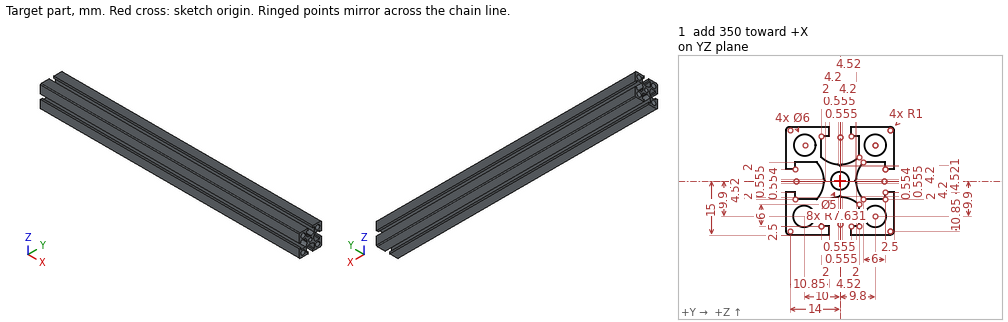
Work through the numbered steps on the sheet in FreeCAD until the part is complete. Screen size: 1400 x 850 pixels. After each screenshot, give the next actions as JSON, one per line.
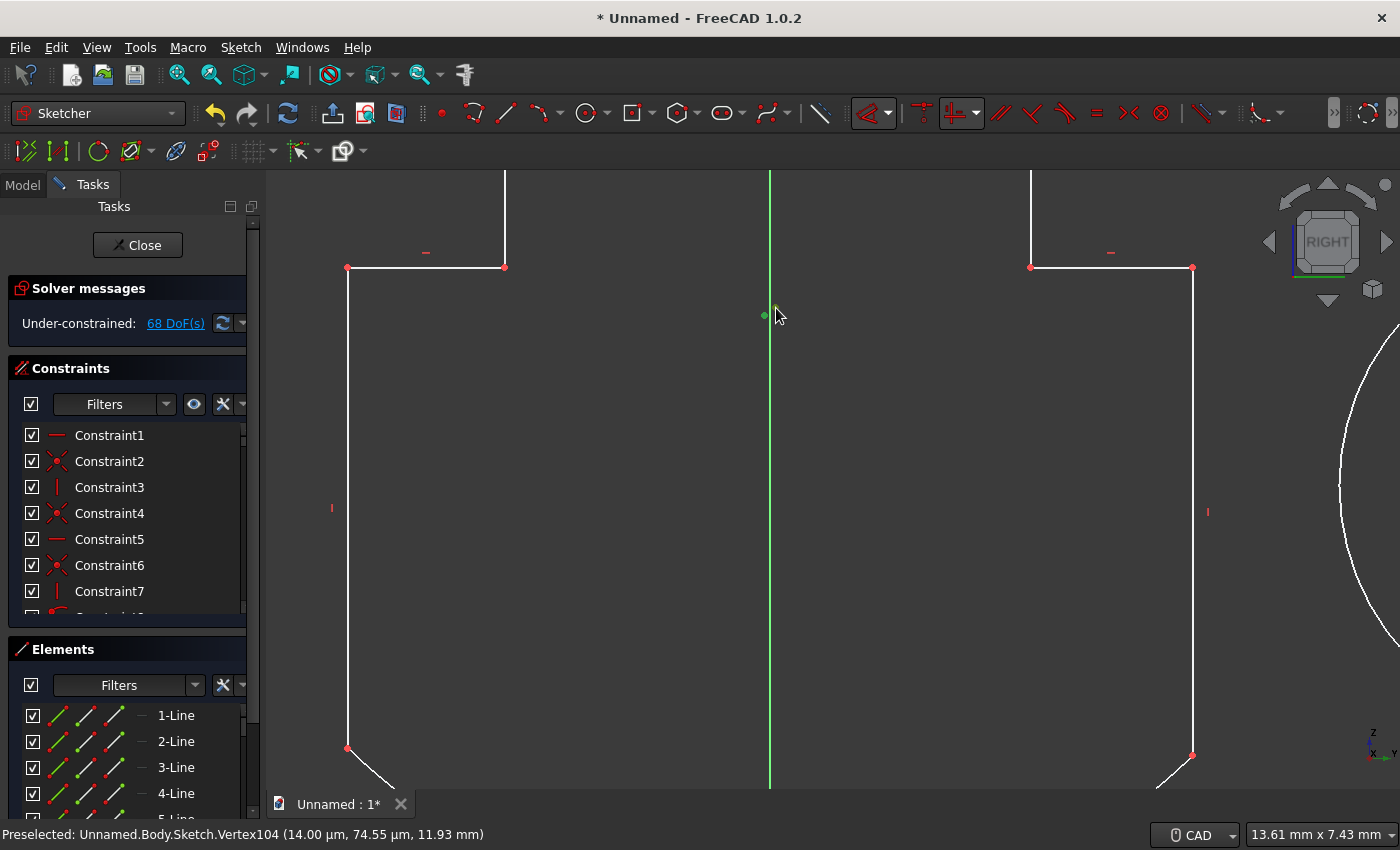
{"action": "left_click", "coordinate": [770, 721]}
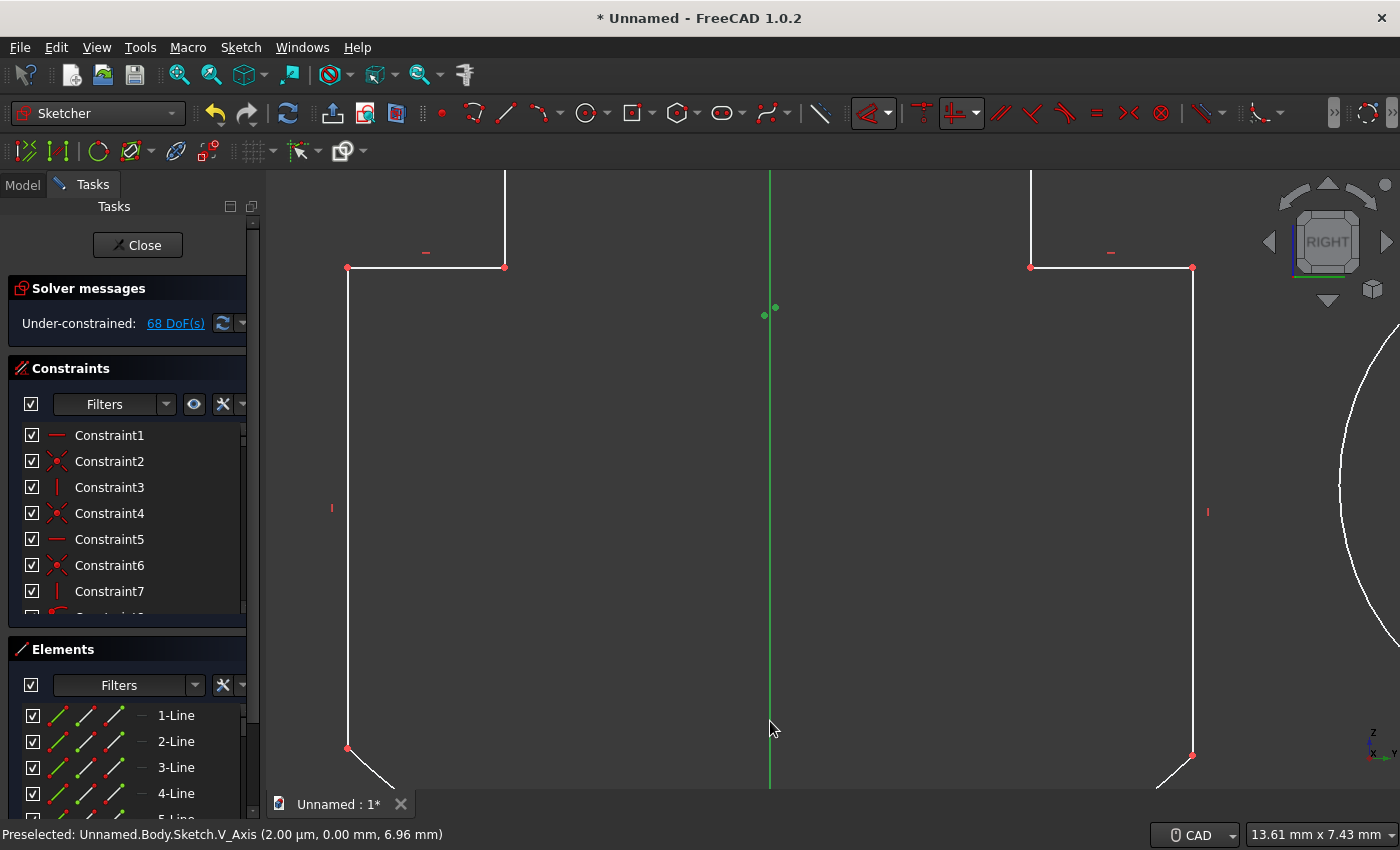
{"action": "left_click", "coordinate": [1130, 114]}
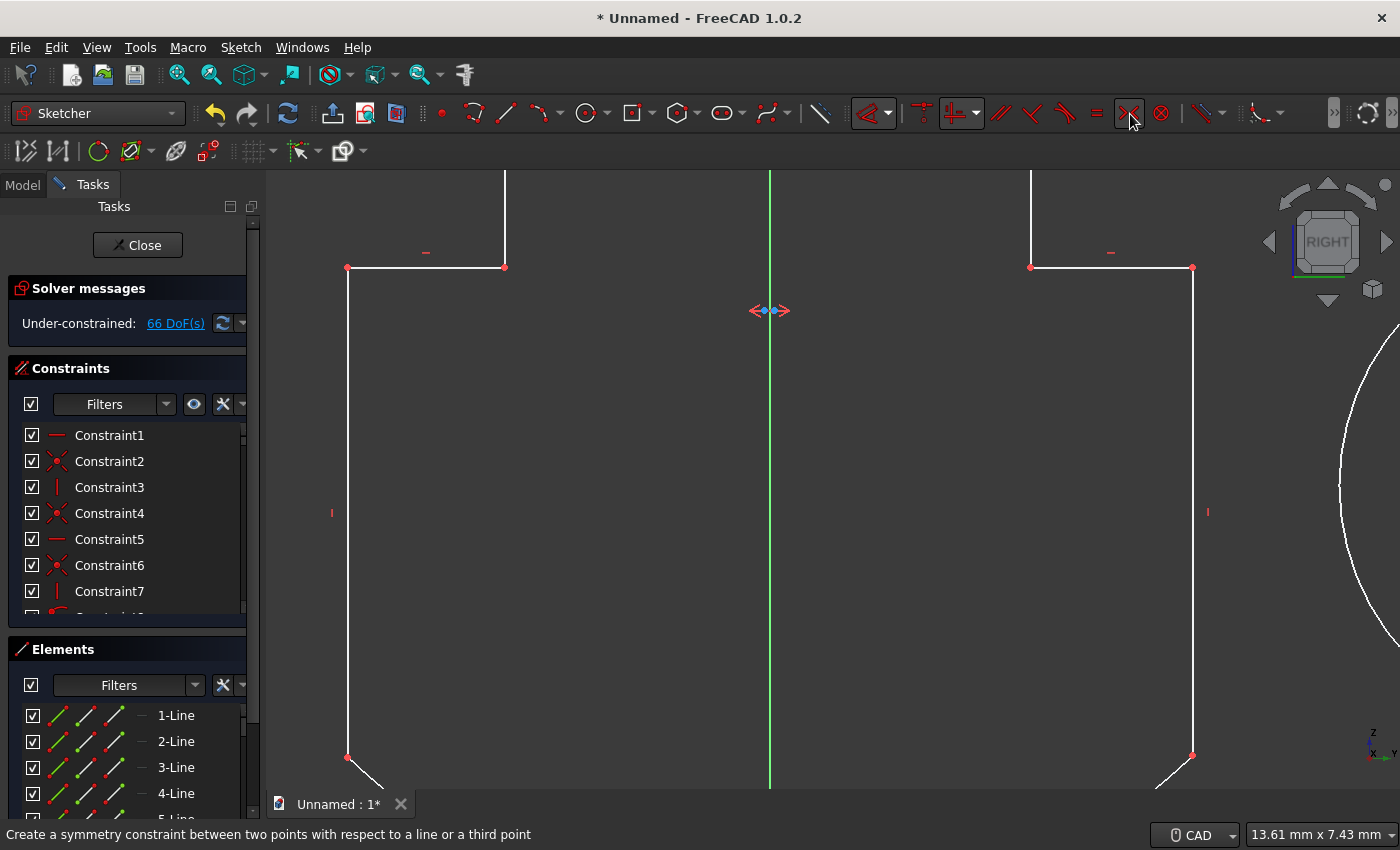
{"action": "scroll", "coordinate": [763, 317], "scroll_direction": "down", "scroll_amount": 9}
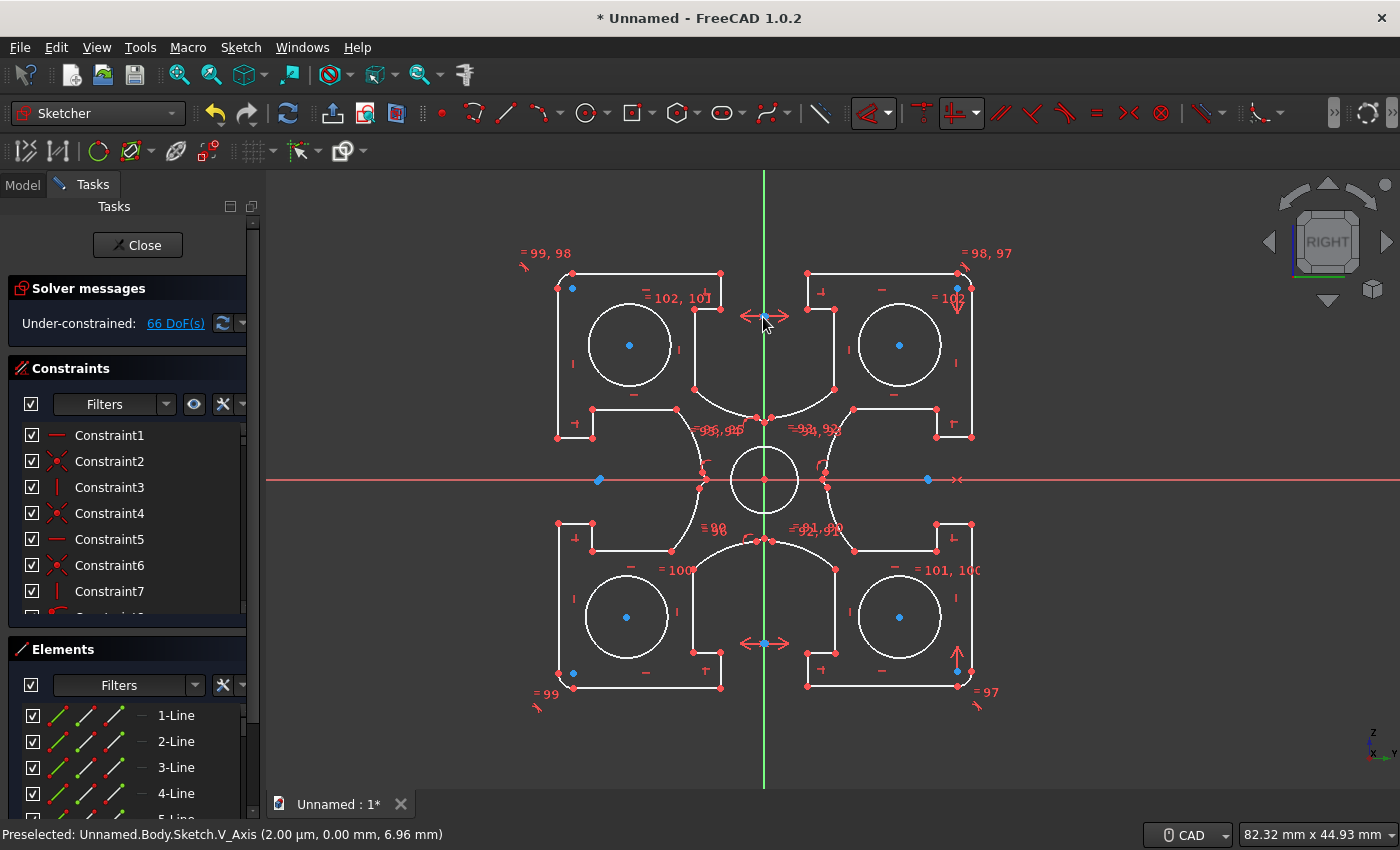
{"action": "left_click", "coordinate": [957, 288]}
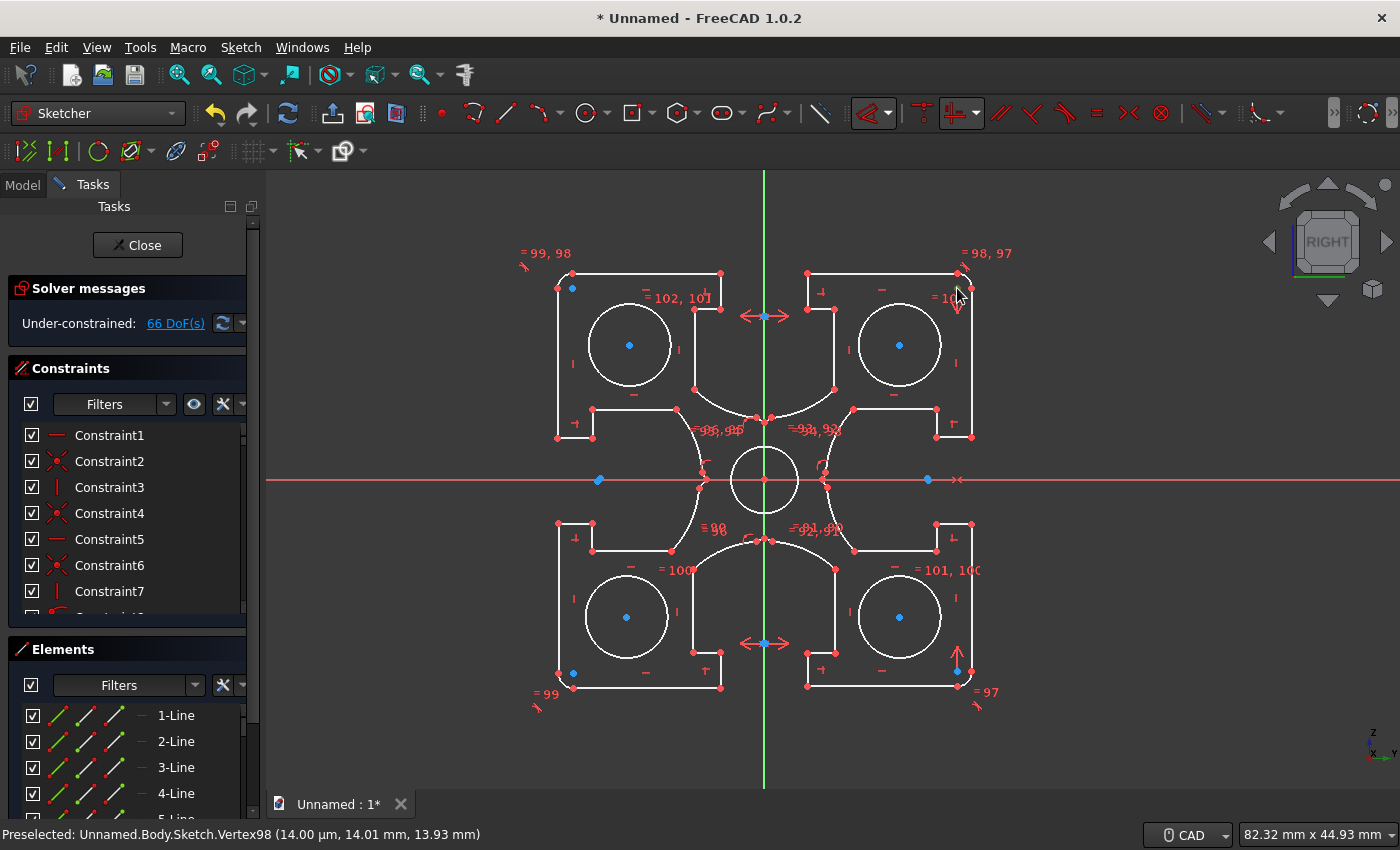
{"action": "left_click", "coordinate": [572, 288]}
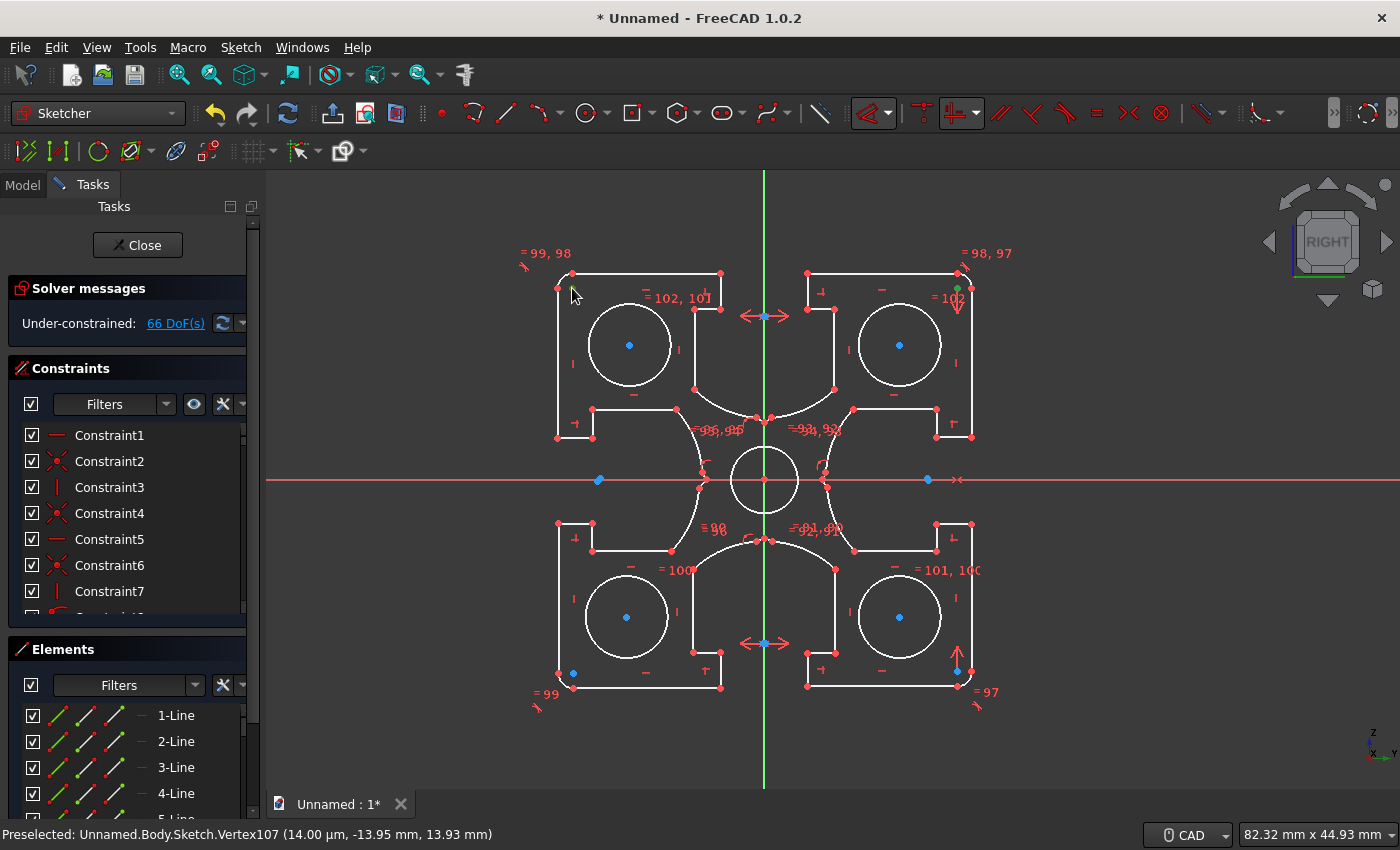
{"action": "left_click", "coordinate": [764, 721]}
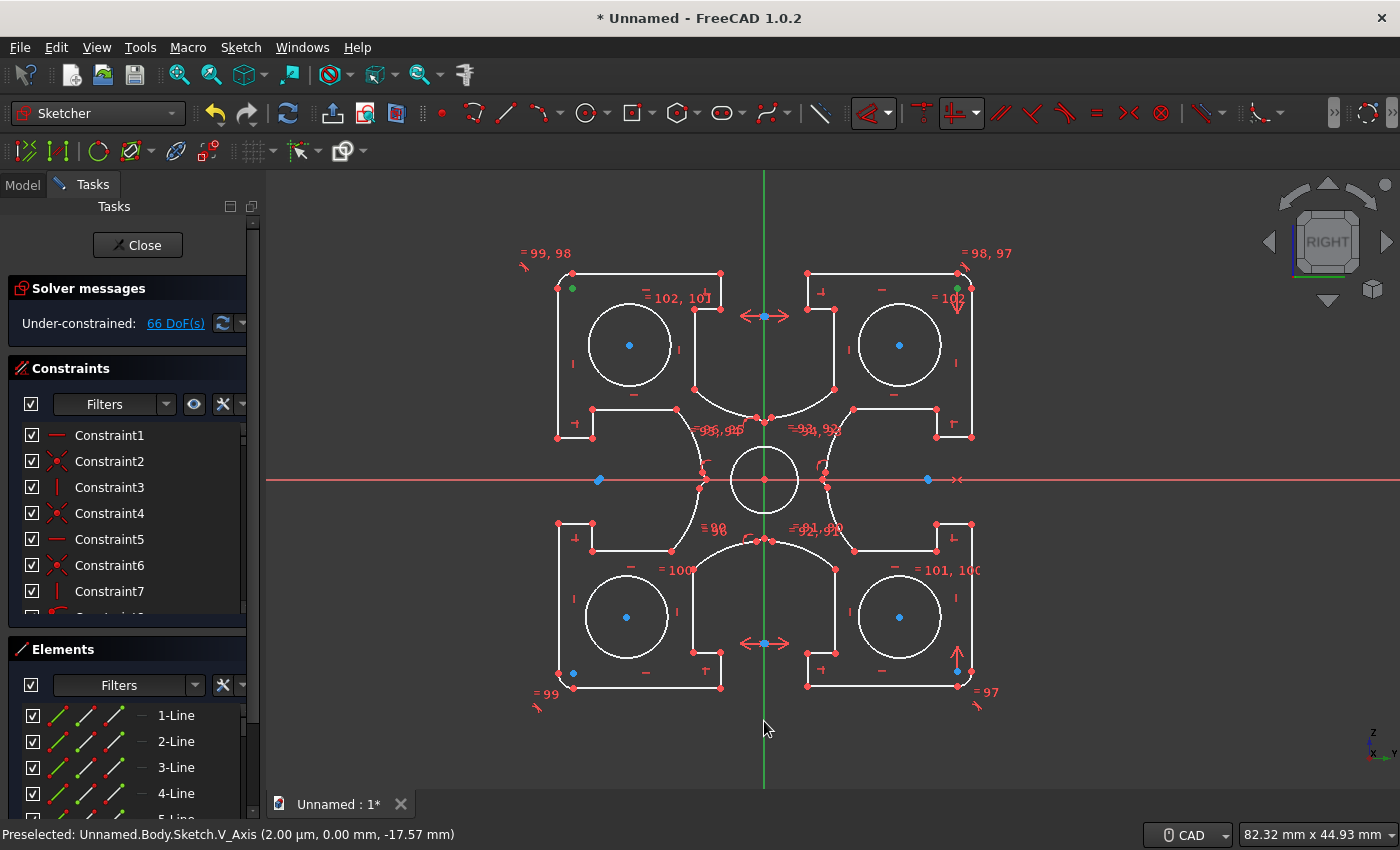
{"action": "key", "text": "s"}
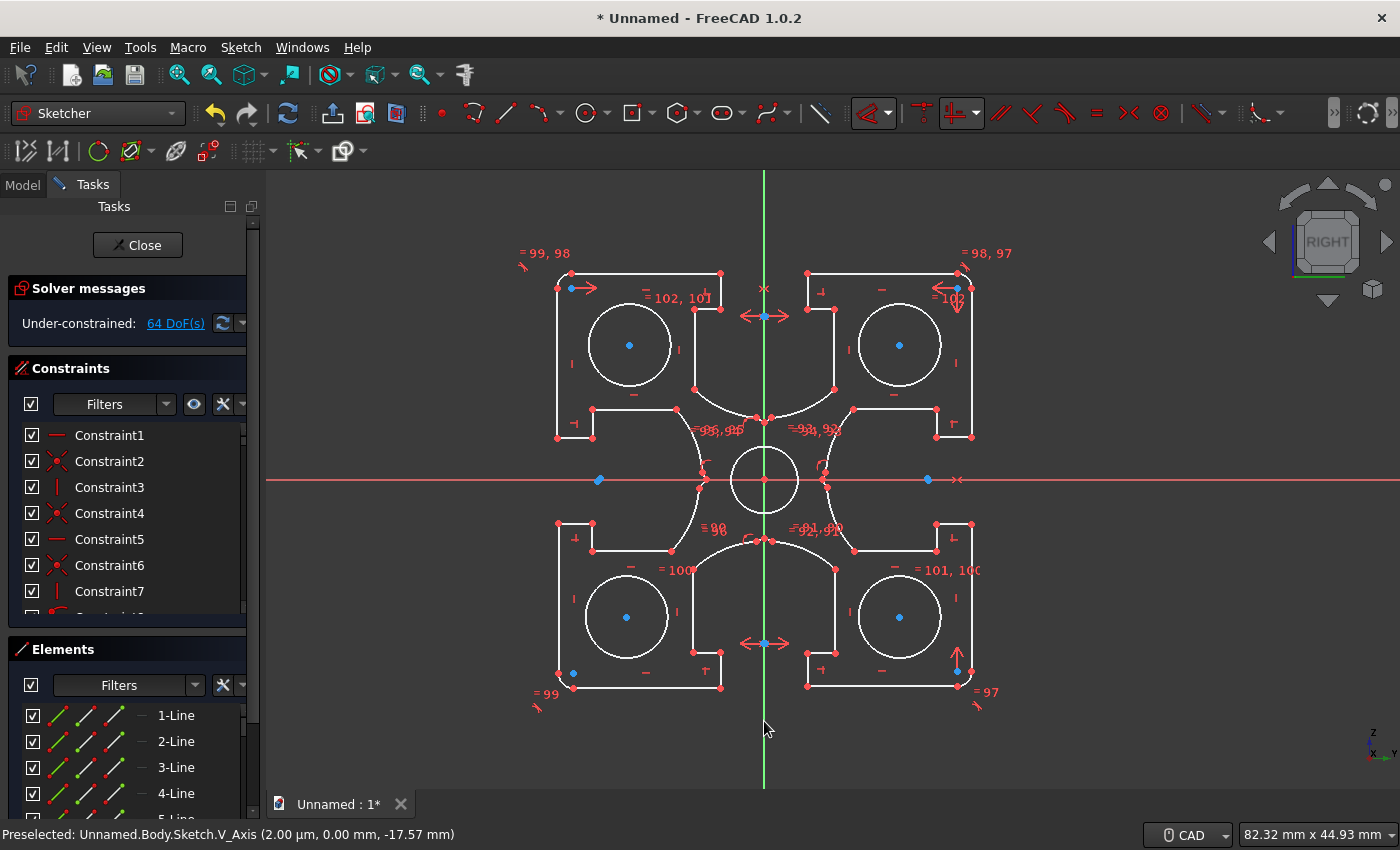
{"action": "scroll", "coordinate": [928, 479], "scroll_direction": "up", "scroll_amount": 9}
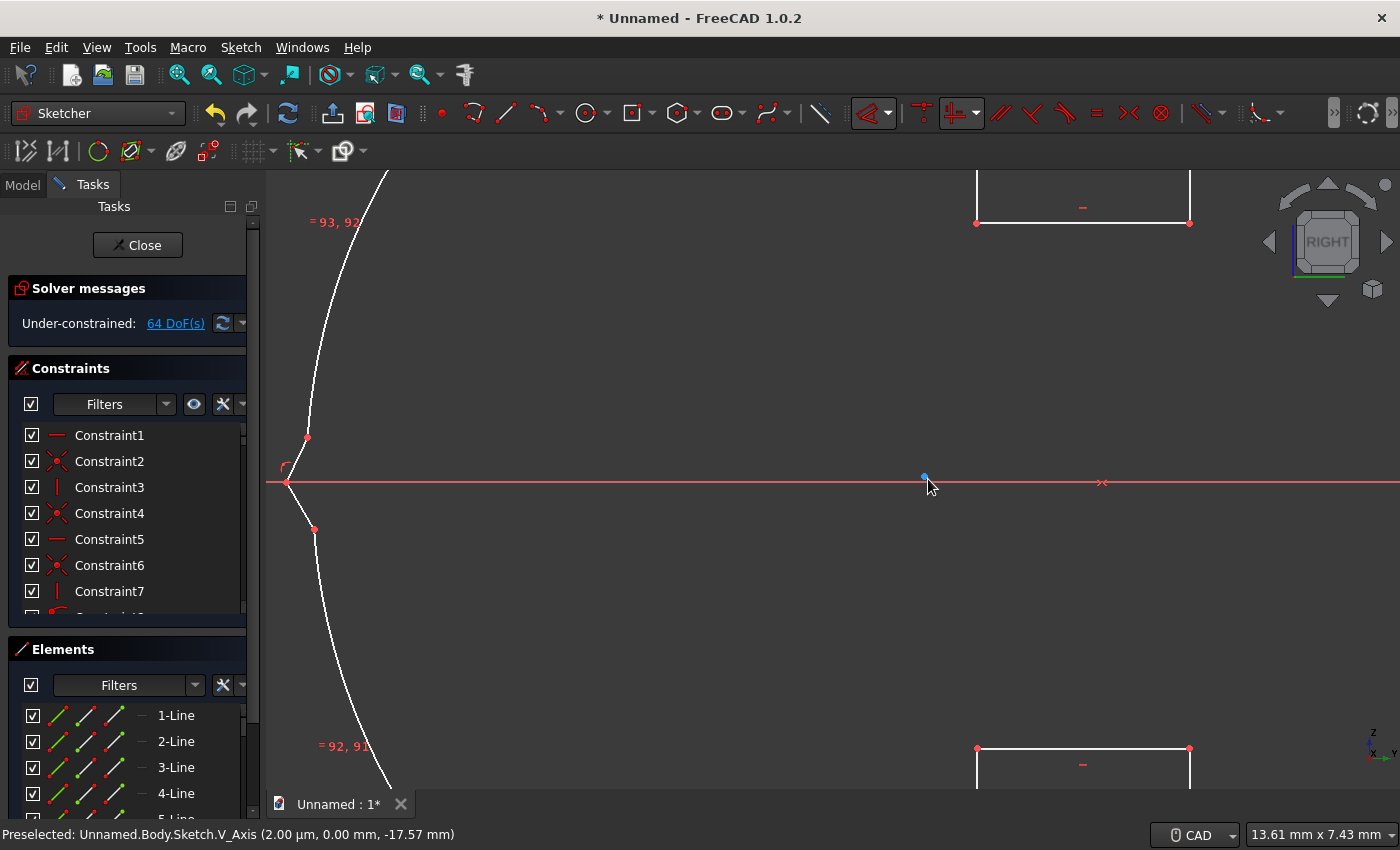
{"action": "left_click", "coordinate": [924, 476]}